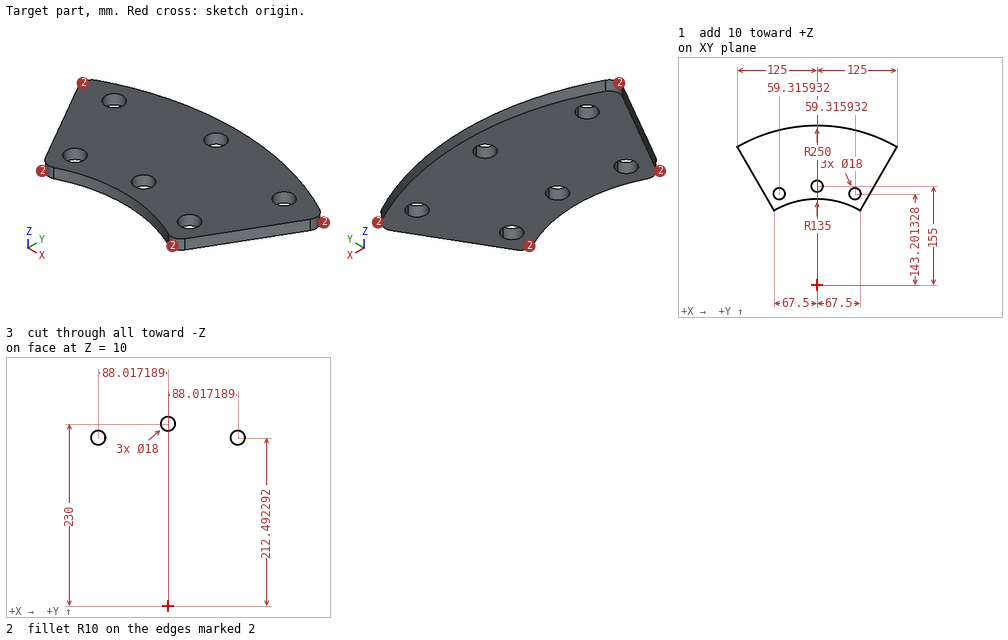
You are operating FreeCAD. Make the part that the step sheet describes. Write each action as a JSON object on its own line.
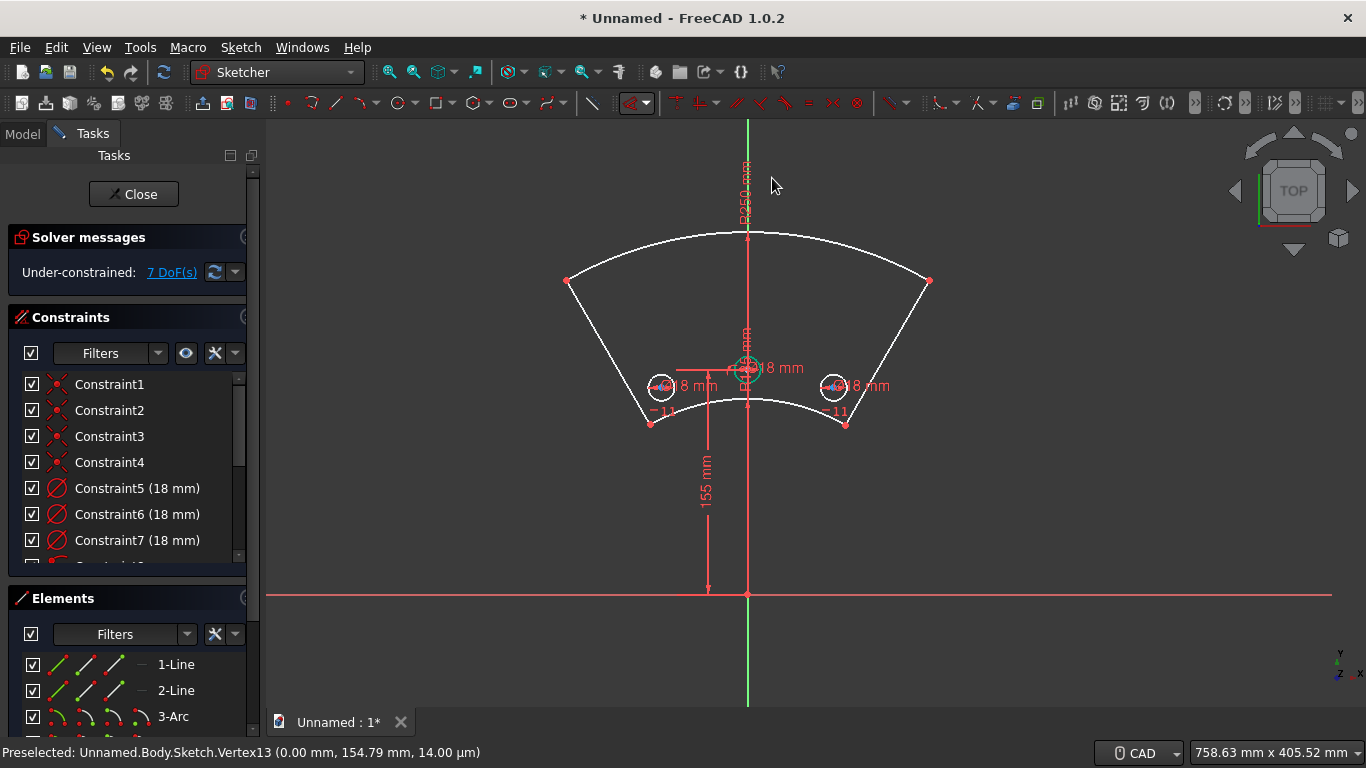
{"action": "left_click", "coordinate": [566, 281]}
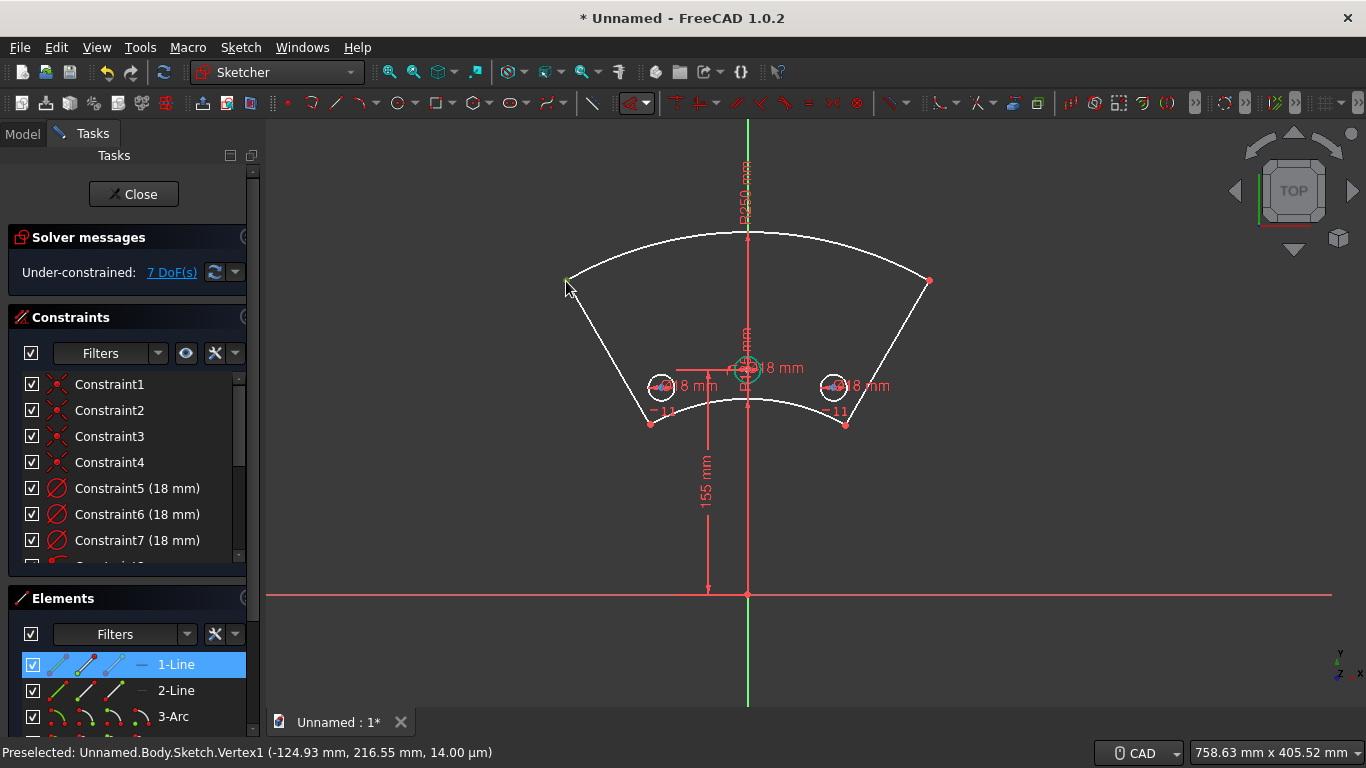
{"action": "left_click", "coordinate": [648, 104]}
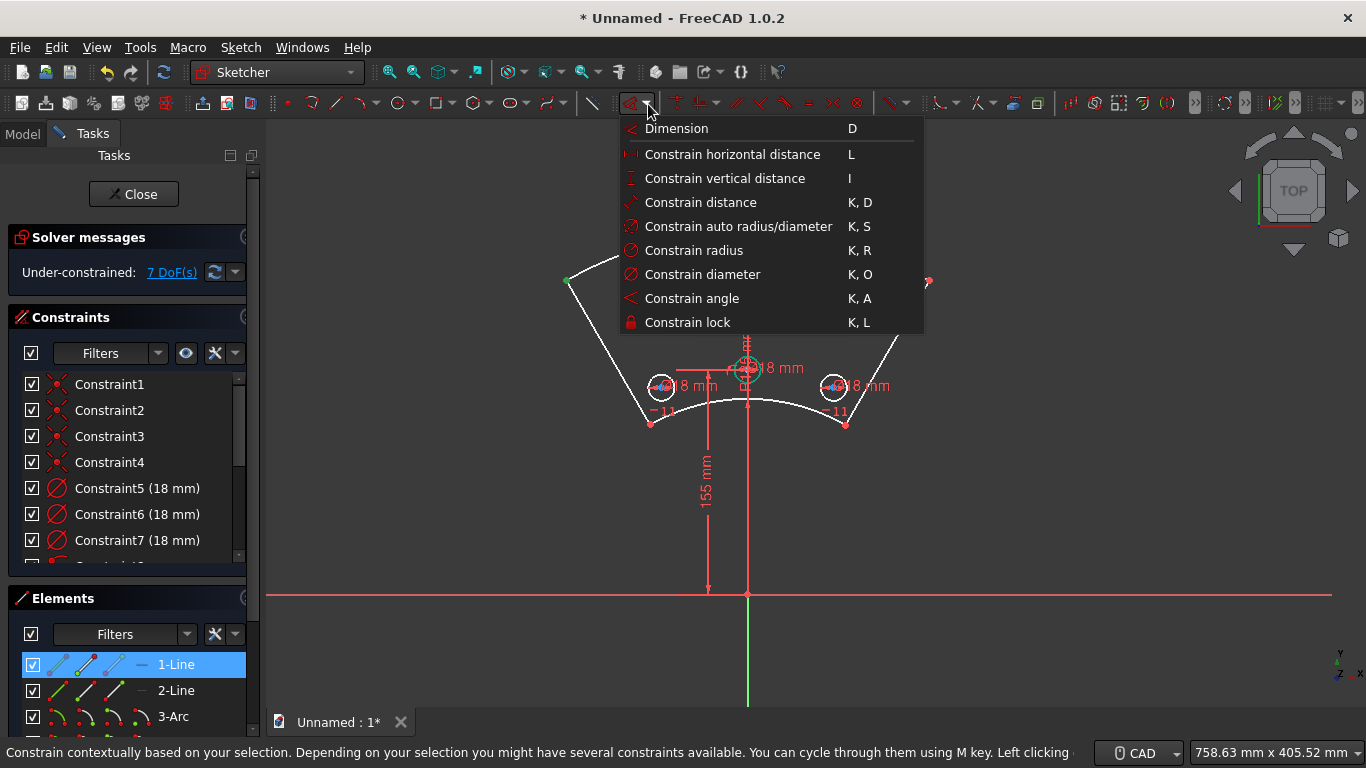
{"action": "left_click", "coordinate": [772, 154]}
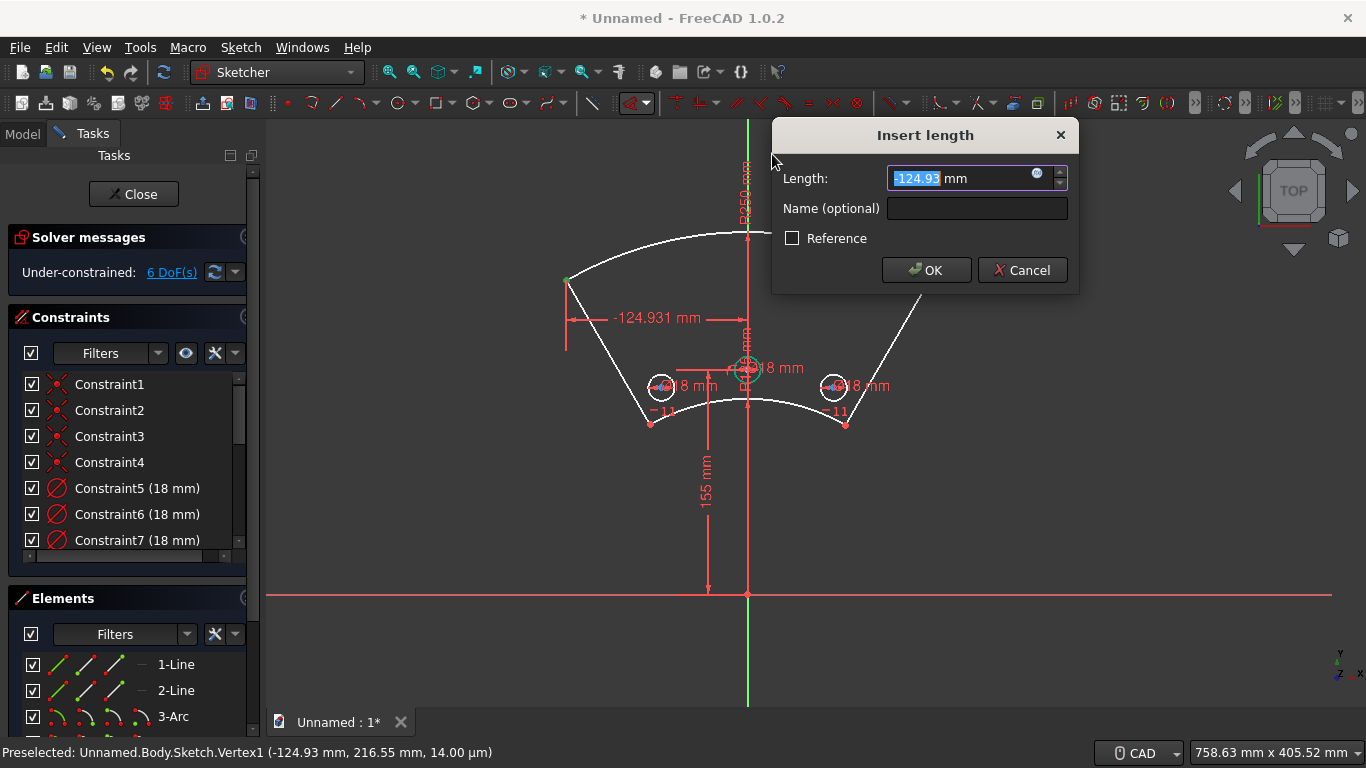
{"action": "type", "text": "-125"}
{"action": "key", "text": "Return"}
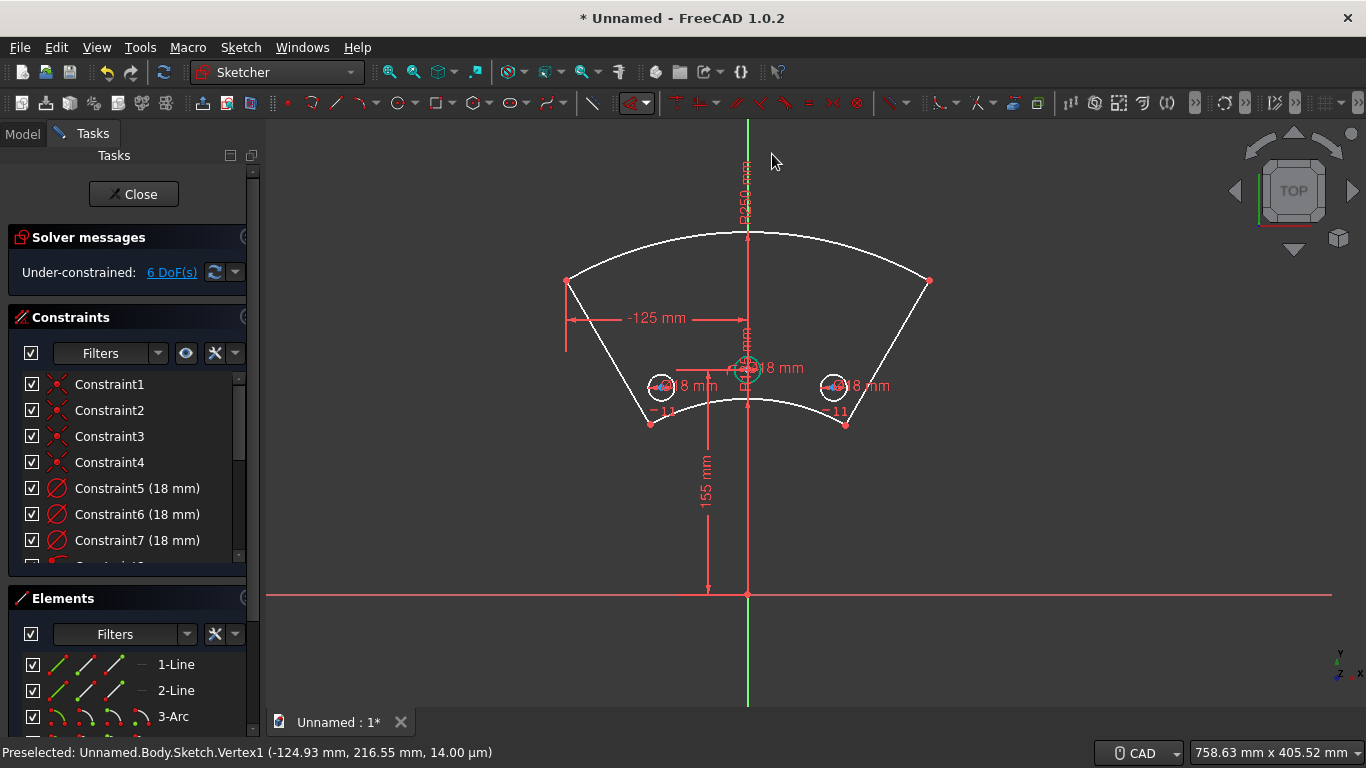
{"action": "left_click", "coordinate": [929, 281]}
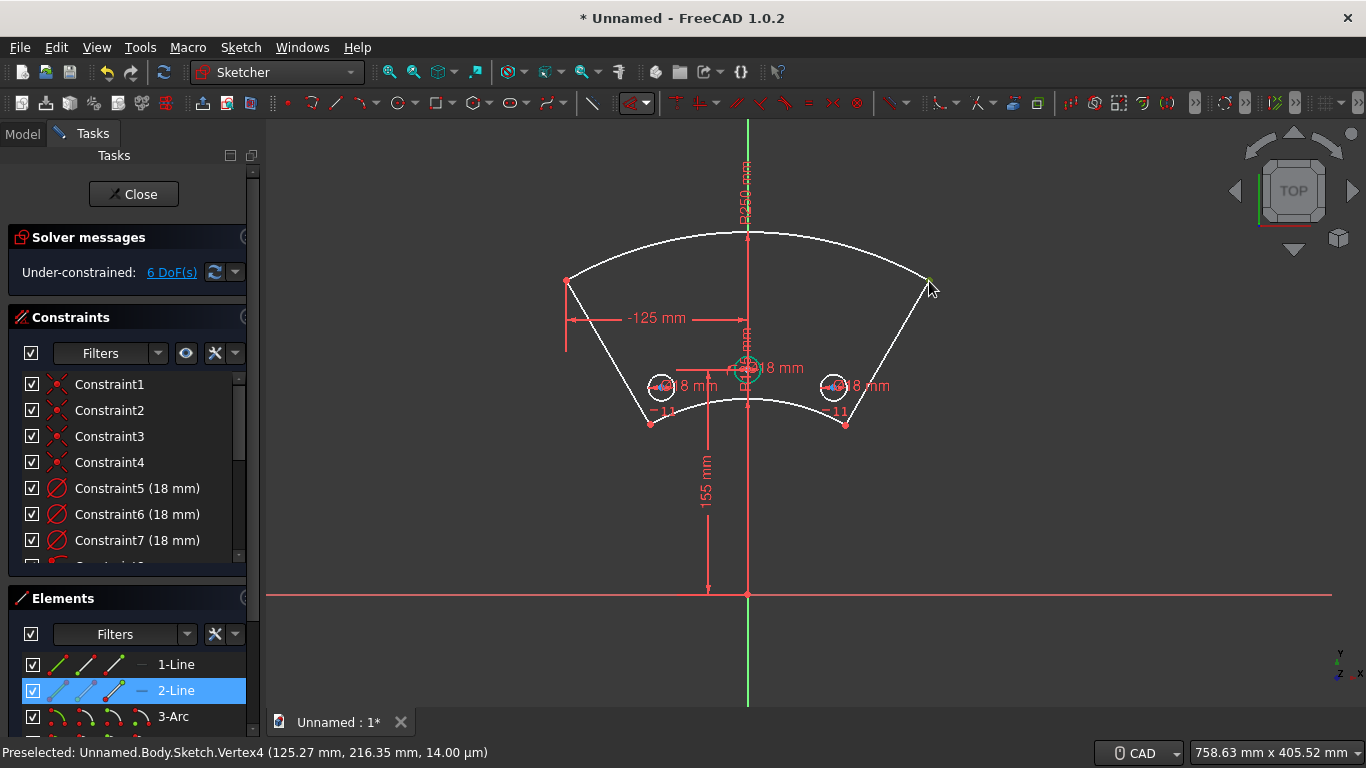
{"action": "left_click", "coordinate": [648, 104]}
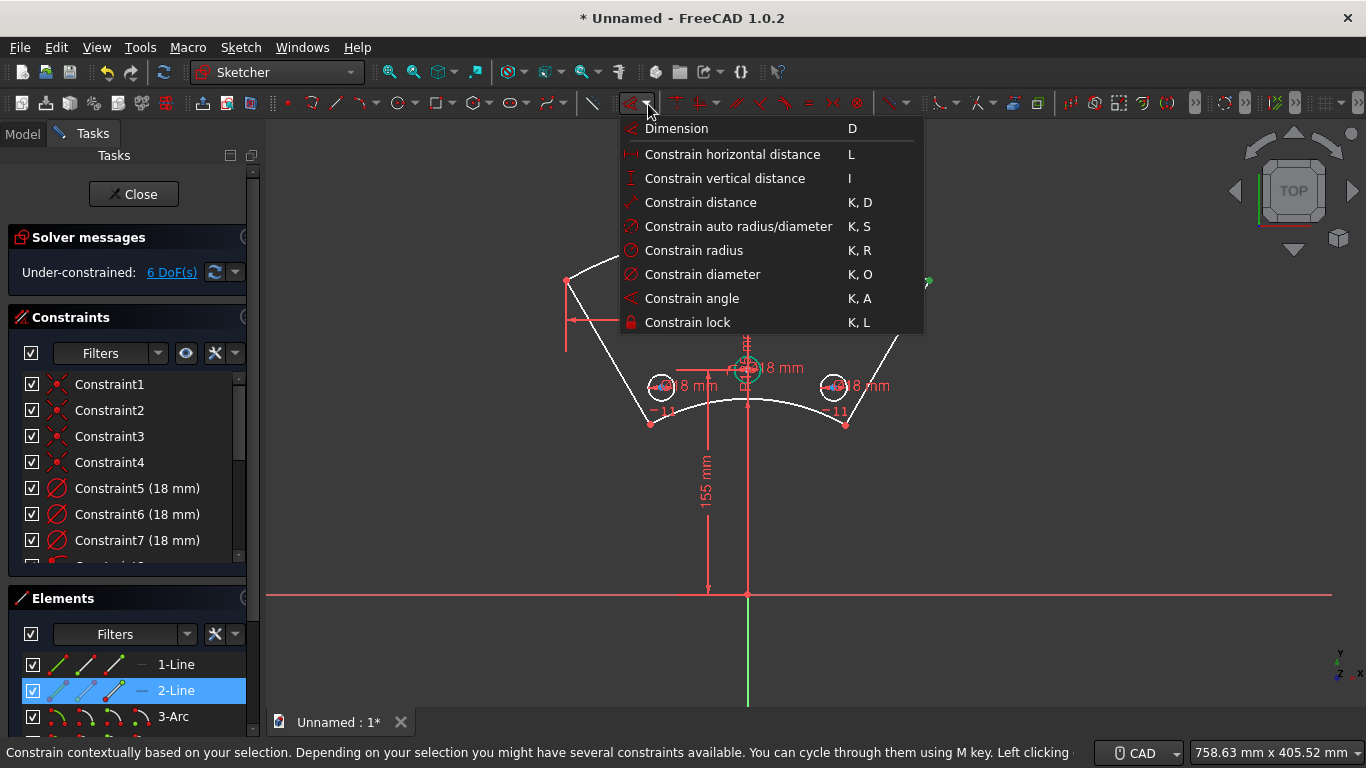
{"action": "left_click", "coordinate": [772, 154]}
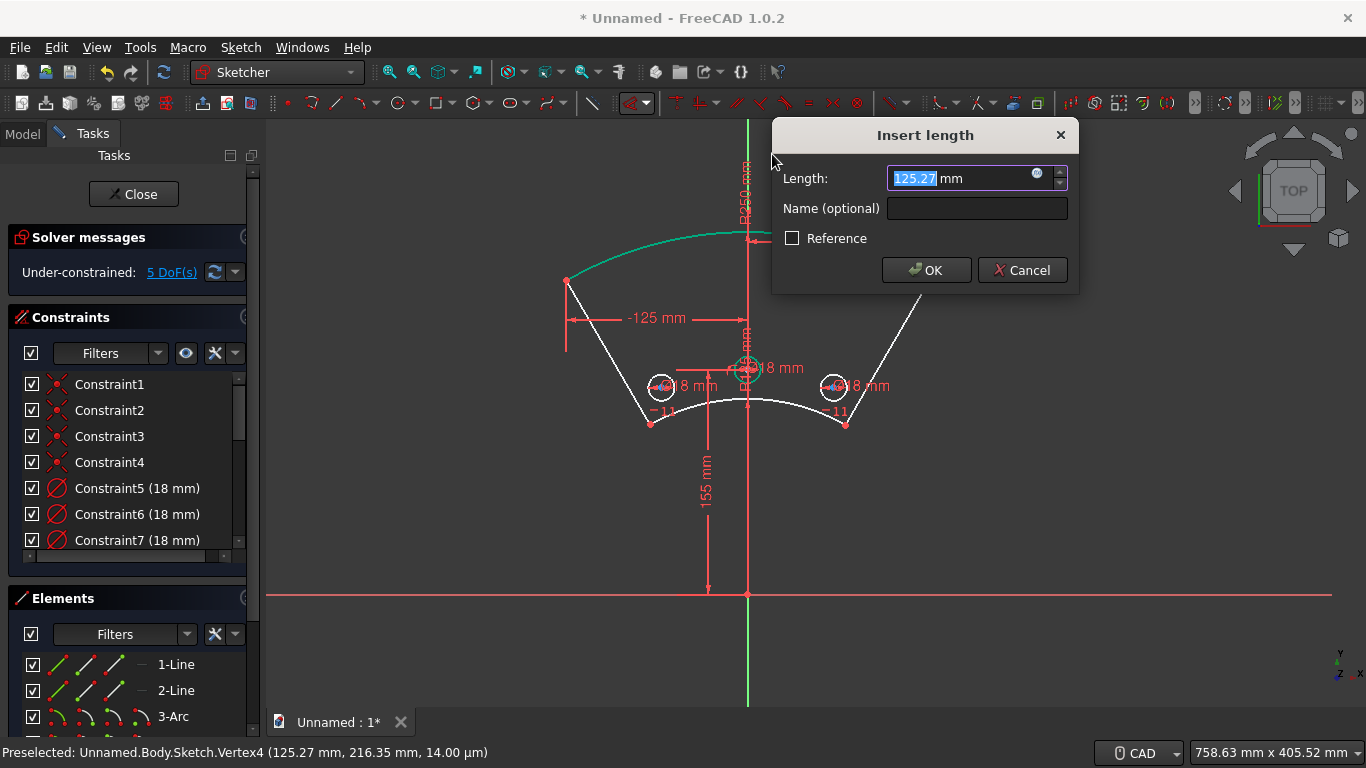
{"action": "type", "text": "125"}
{"action": "key", "text": "Return"}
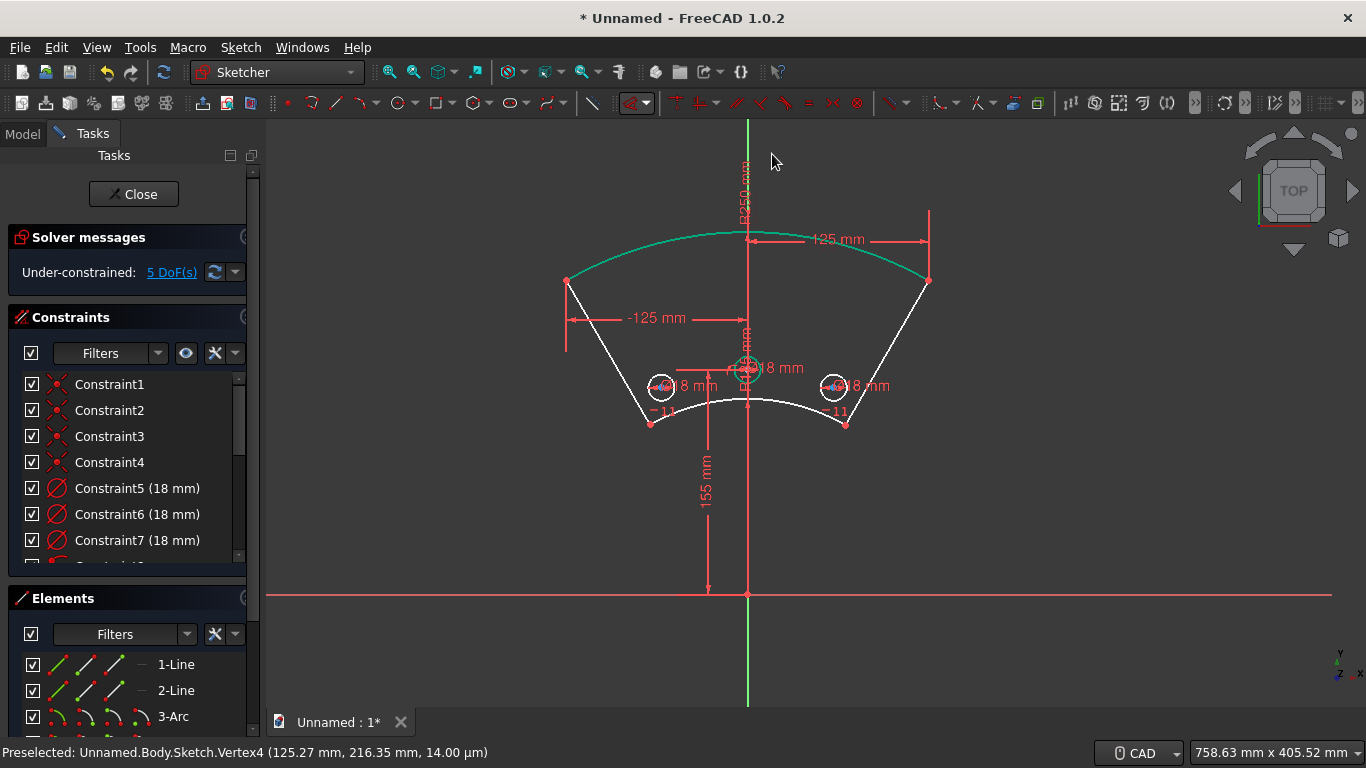
{"action": "left_click", "coordinate": [650, 425]}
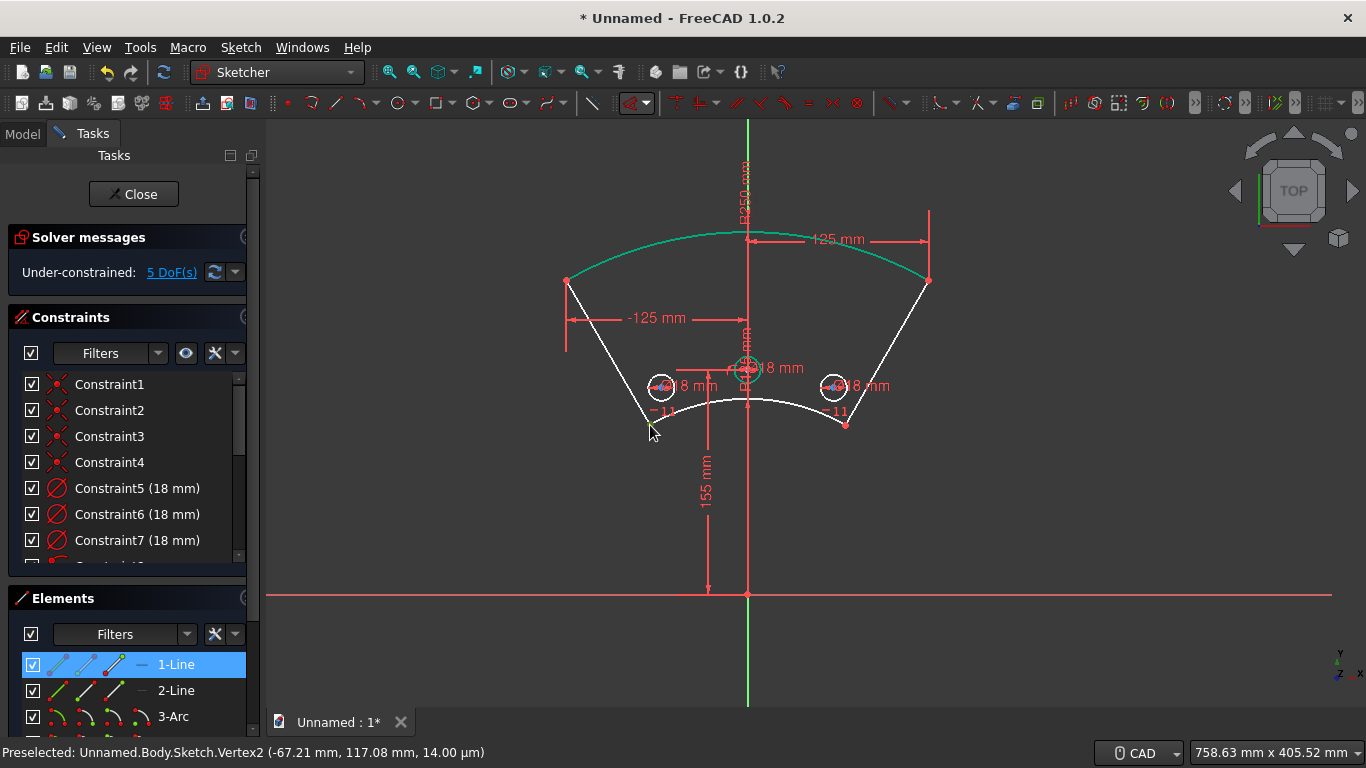
{"action": "key", "text": "l"}